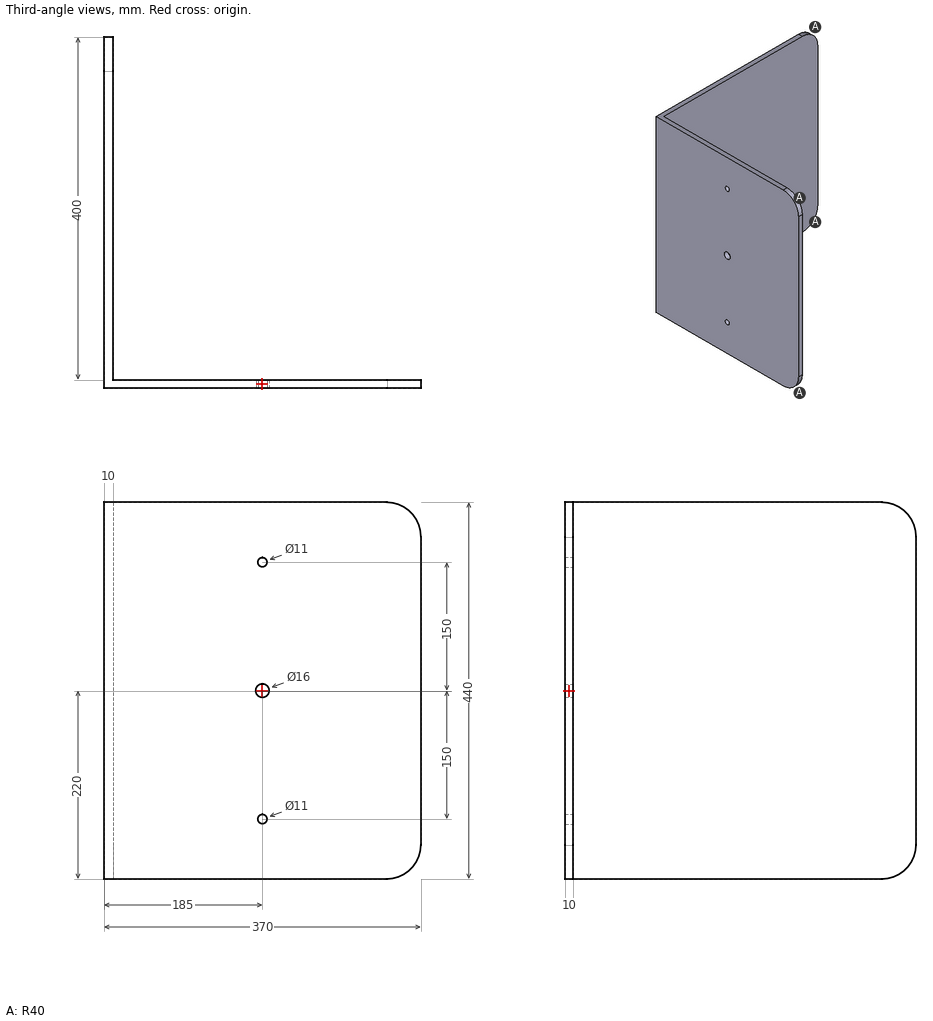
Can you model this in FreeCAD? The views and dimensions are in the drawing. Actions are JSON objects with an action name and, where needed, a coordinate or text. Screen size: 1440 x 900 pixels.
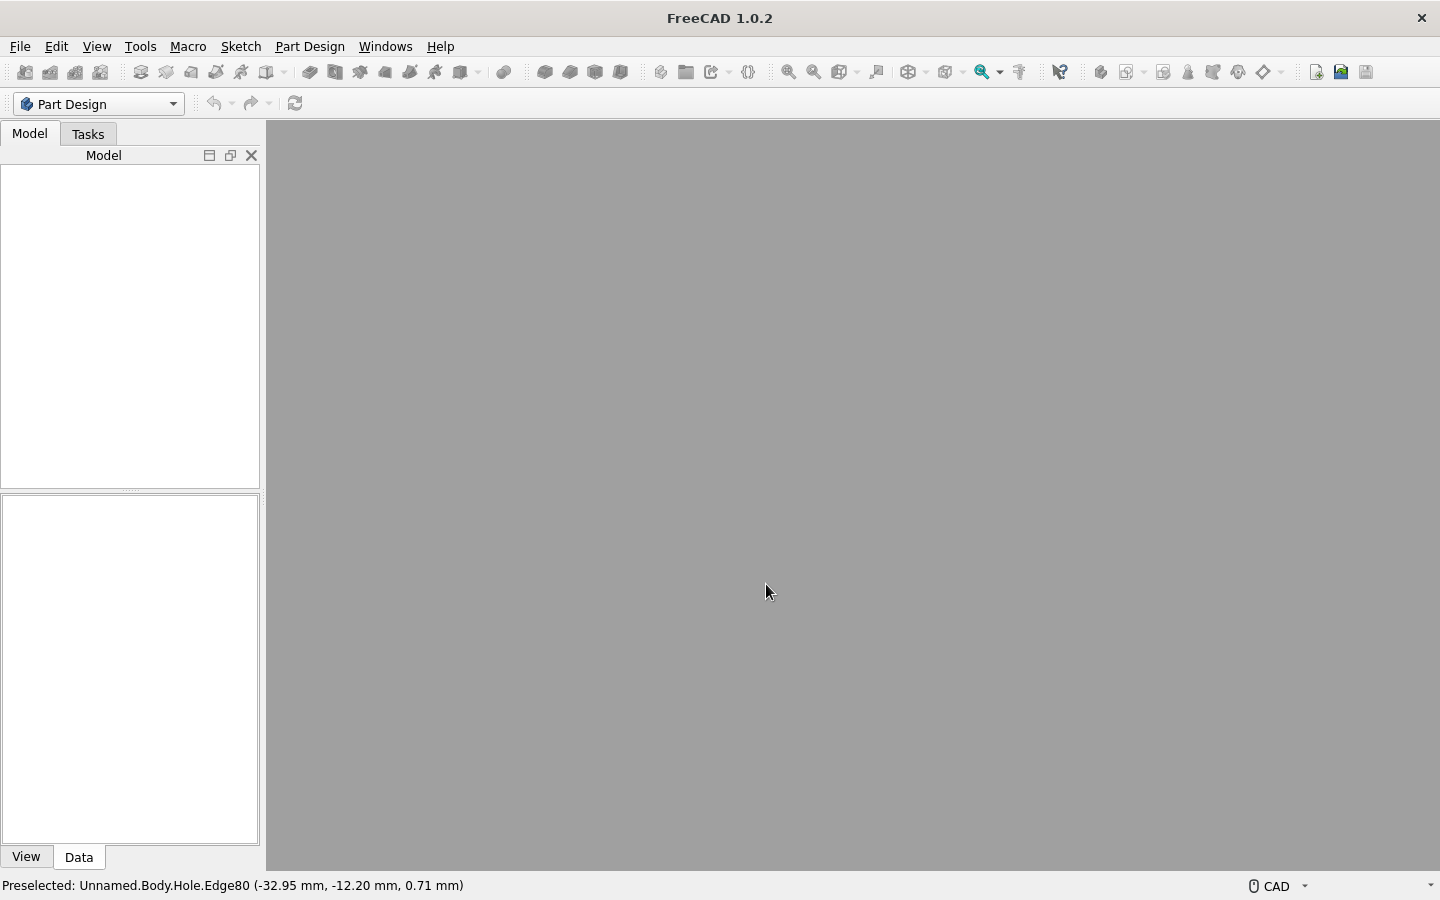
{"action": "left_click", "coordinate": [1316, 72]}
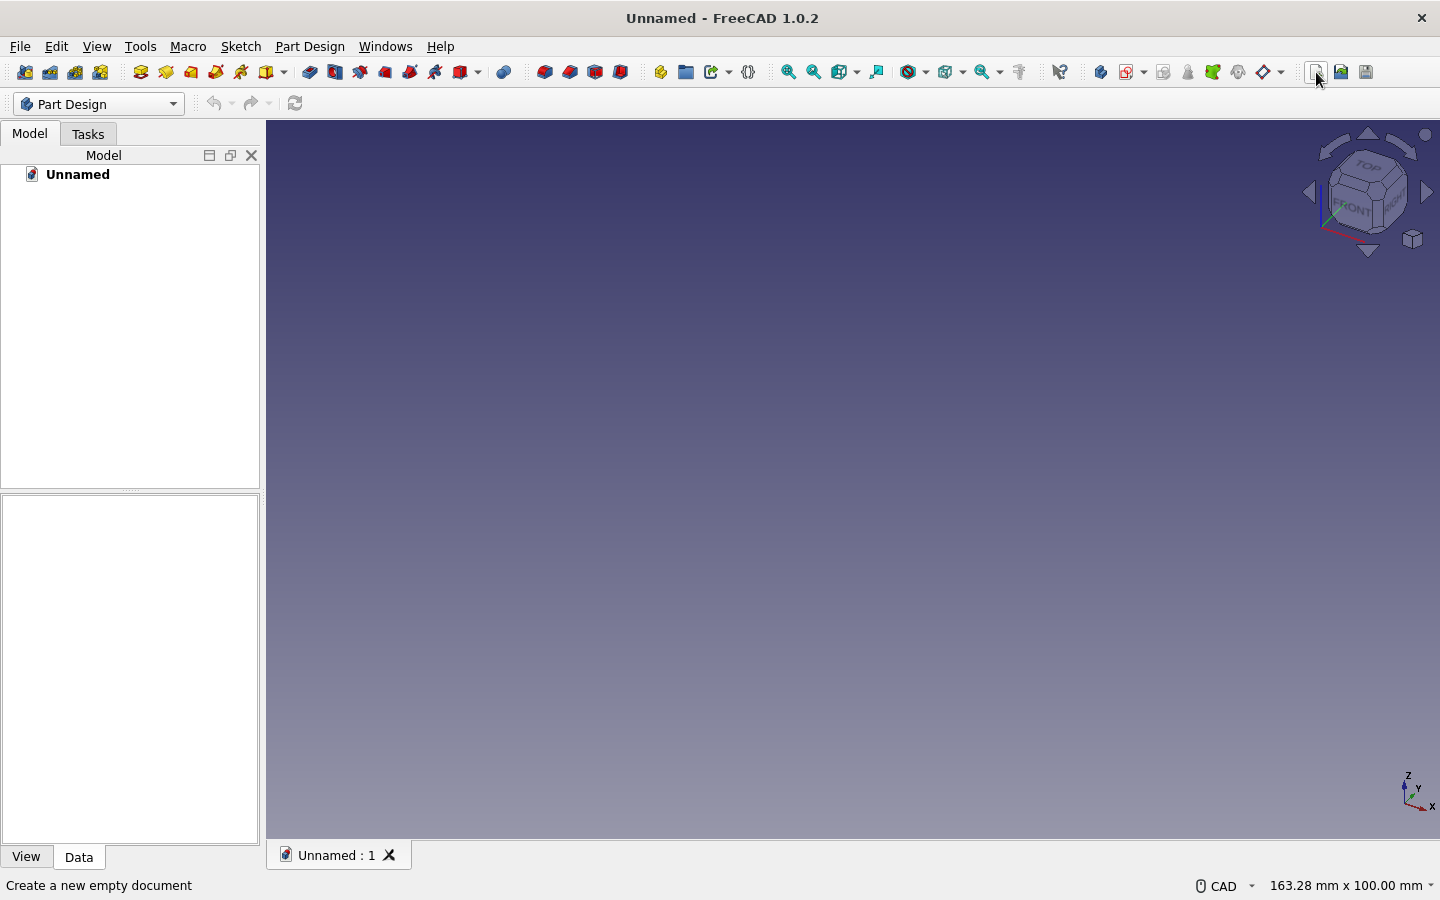
{"action": "left_click", "coordinate": [1126, 72]}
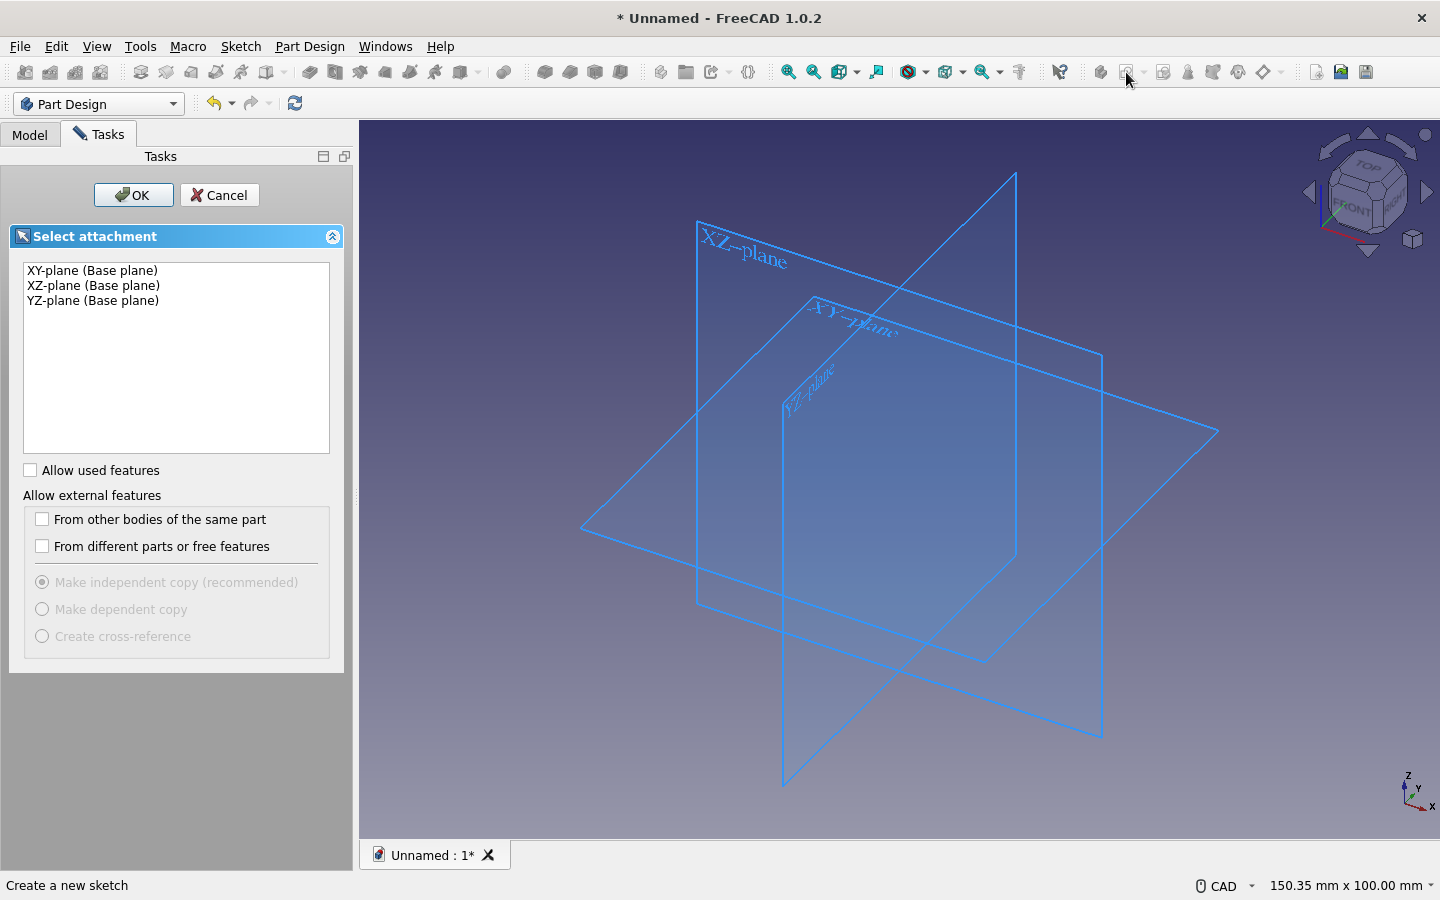
{"action": "left_click", "coordinate": [84, 286]}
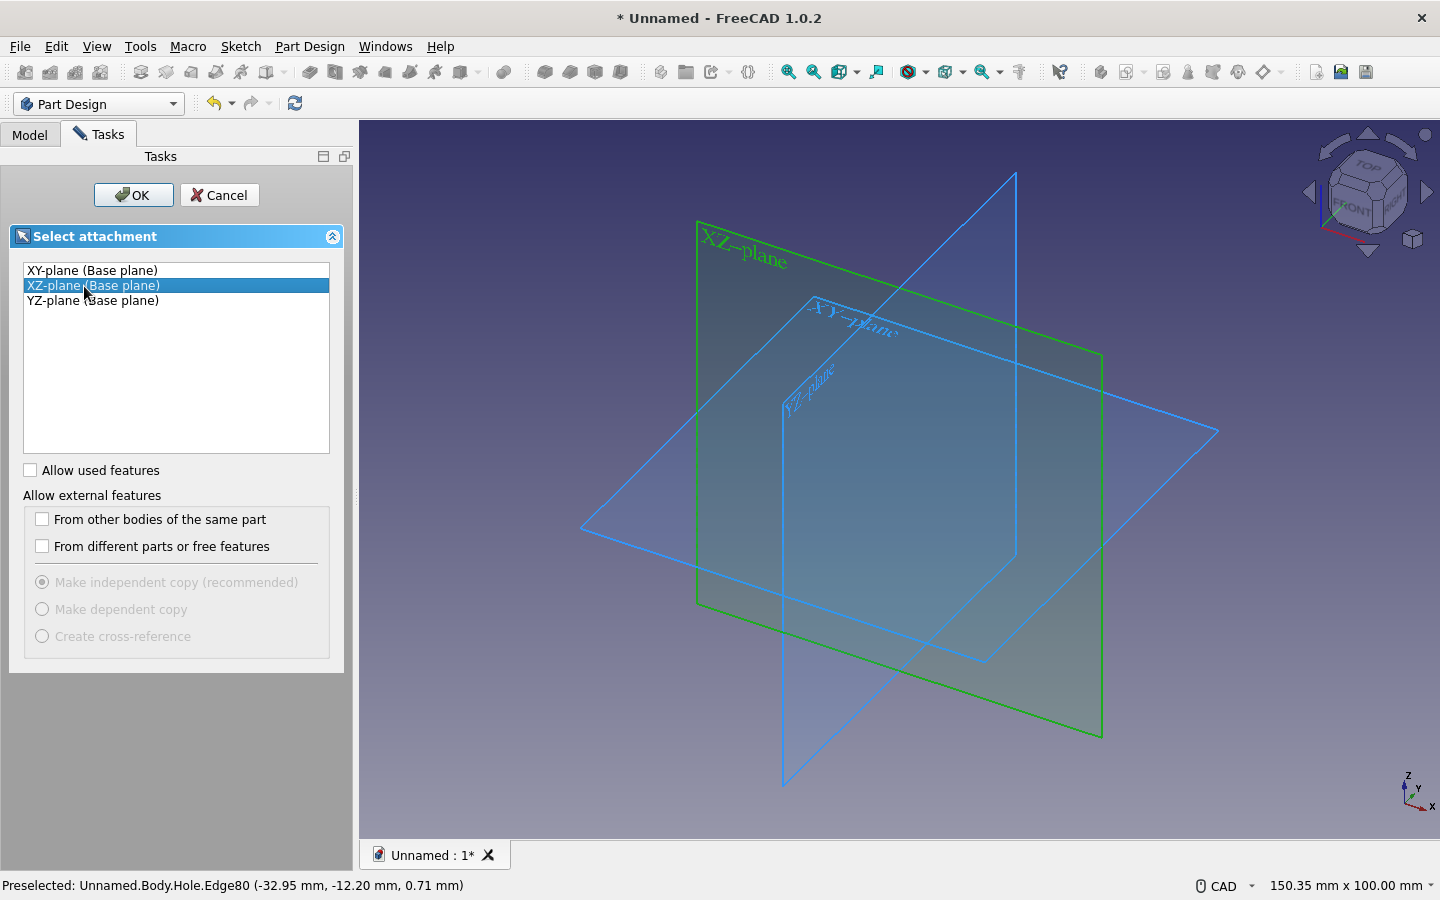
{"action": "left_click", "coordinate": [134, 195]}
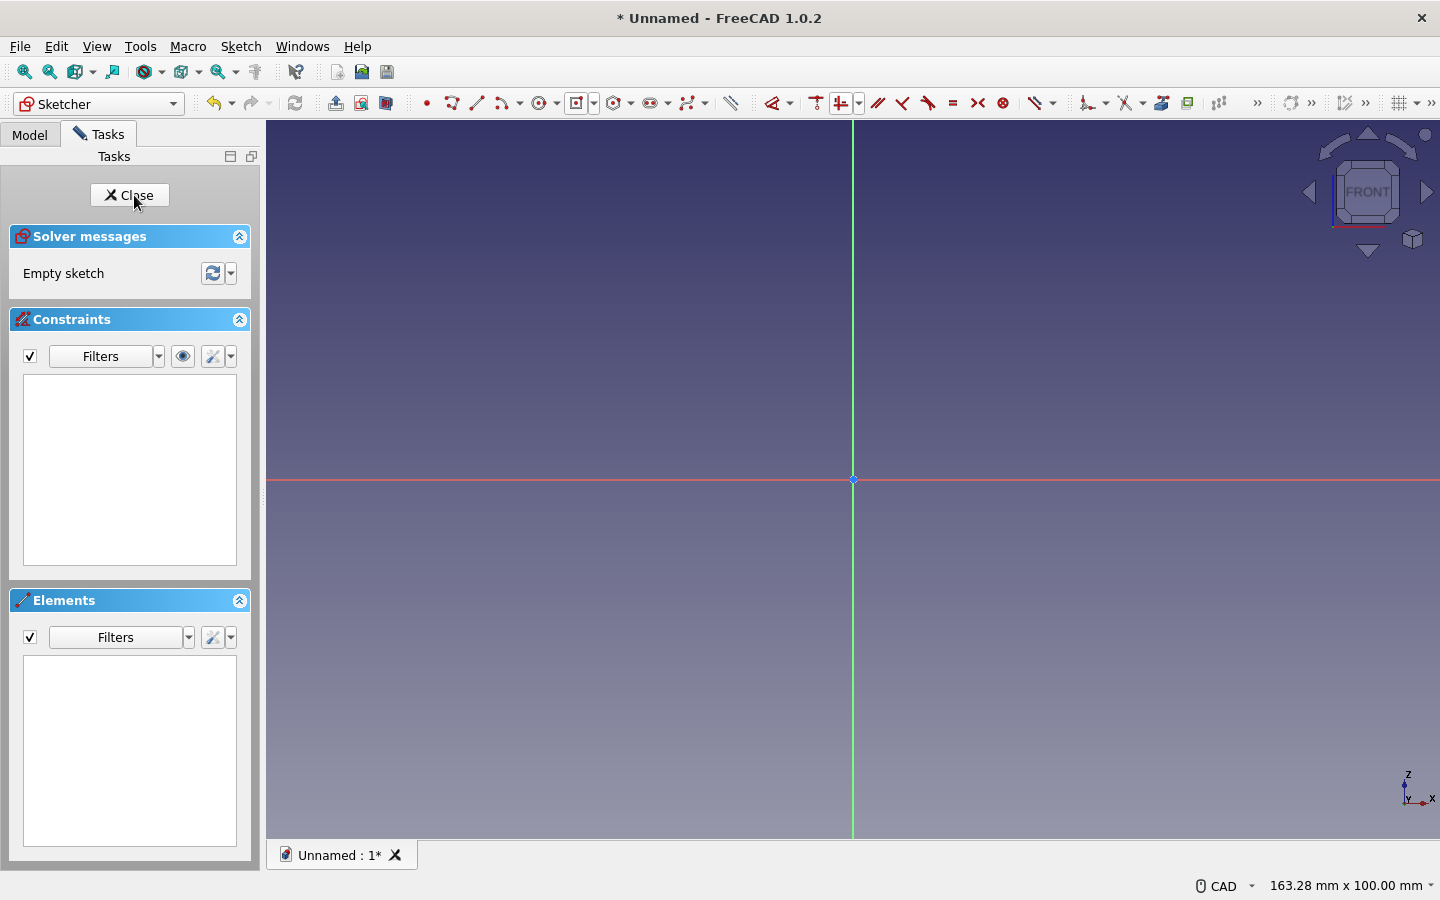
{"action": "scroll", "coordinate": [774, 480], "scroll_direction": "down", "scroll_amount": 10}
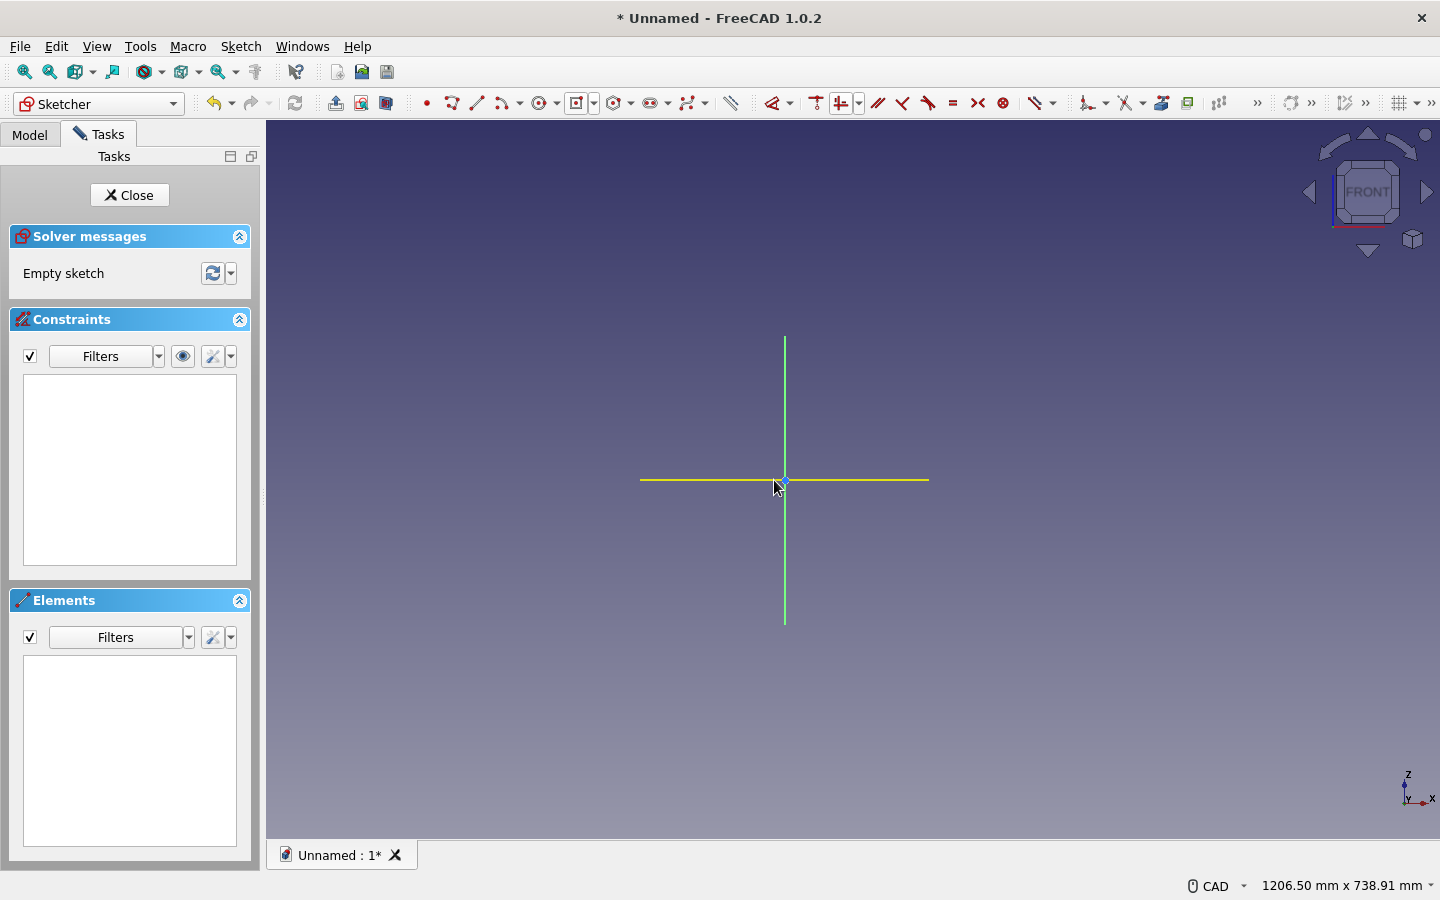
{"action": "left_click", "coordinate": [576, 104]}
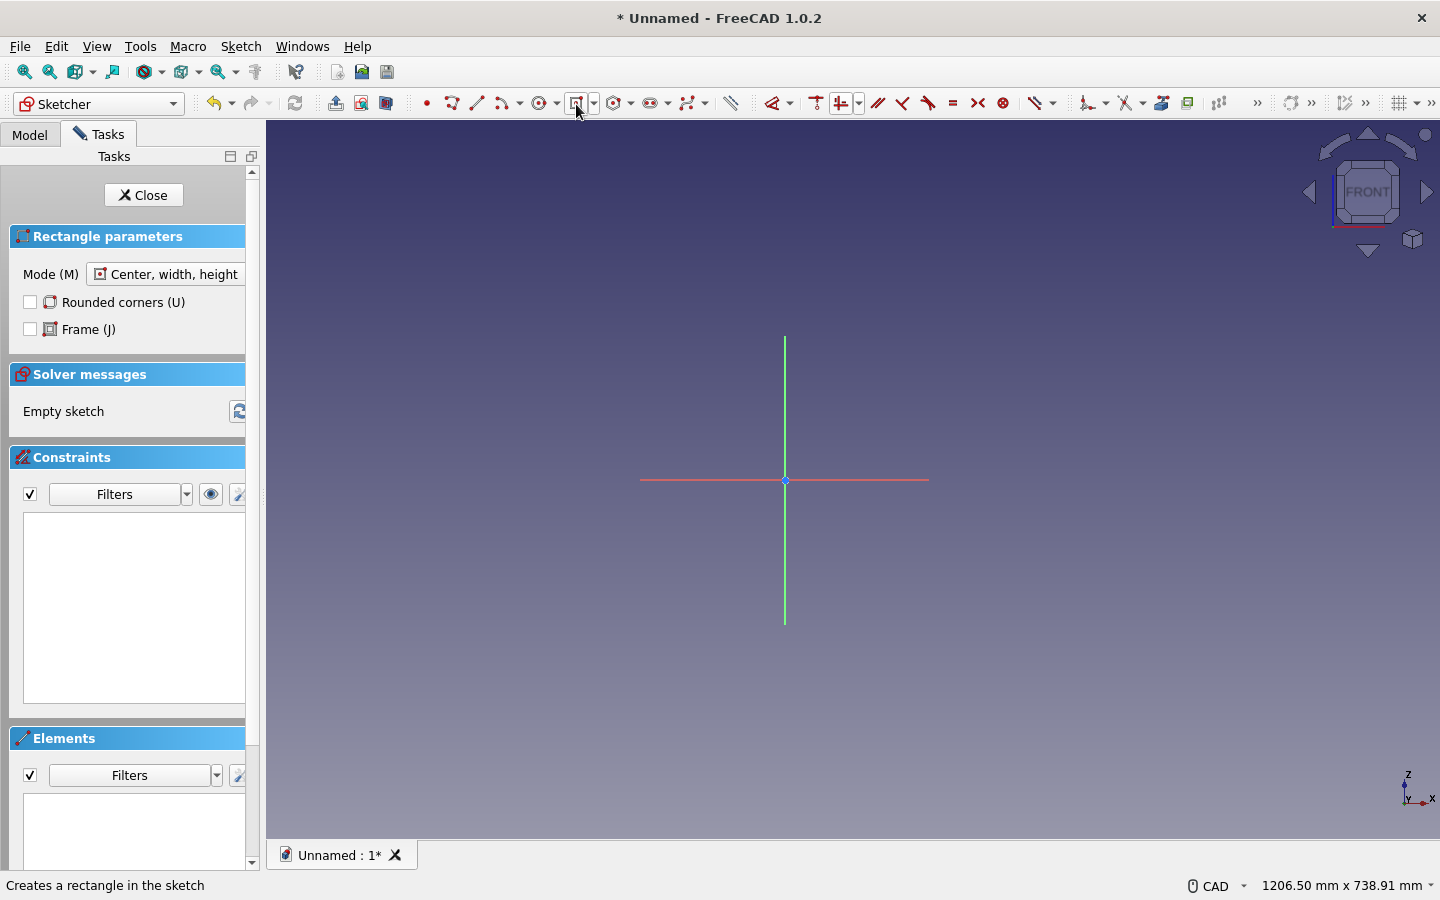
{"action": "left_click", "coordinate": [785, 480]}
{"action": "mouse_move", "coordinate": [965, 266]}